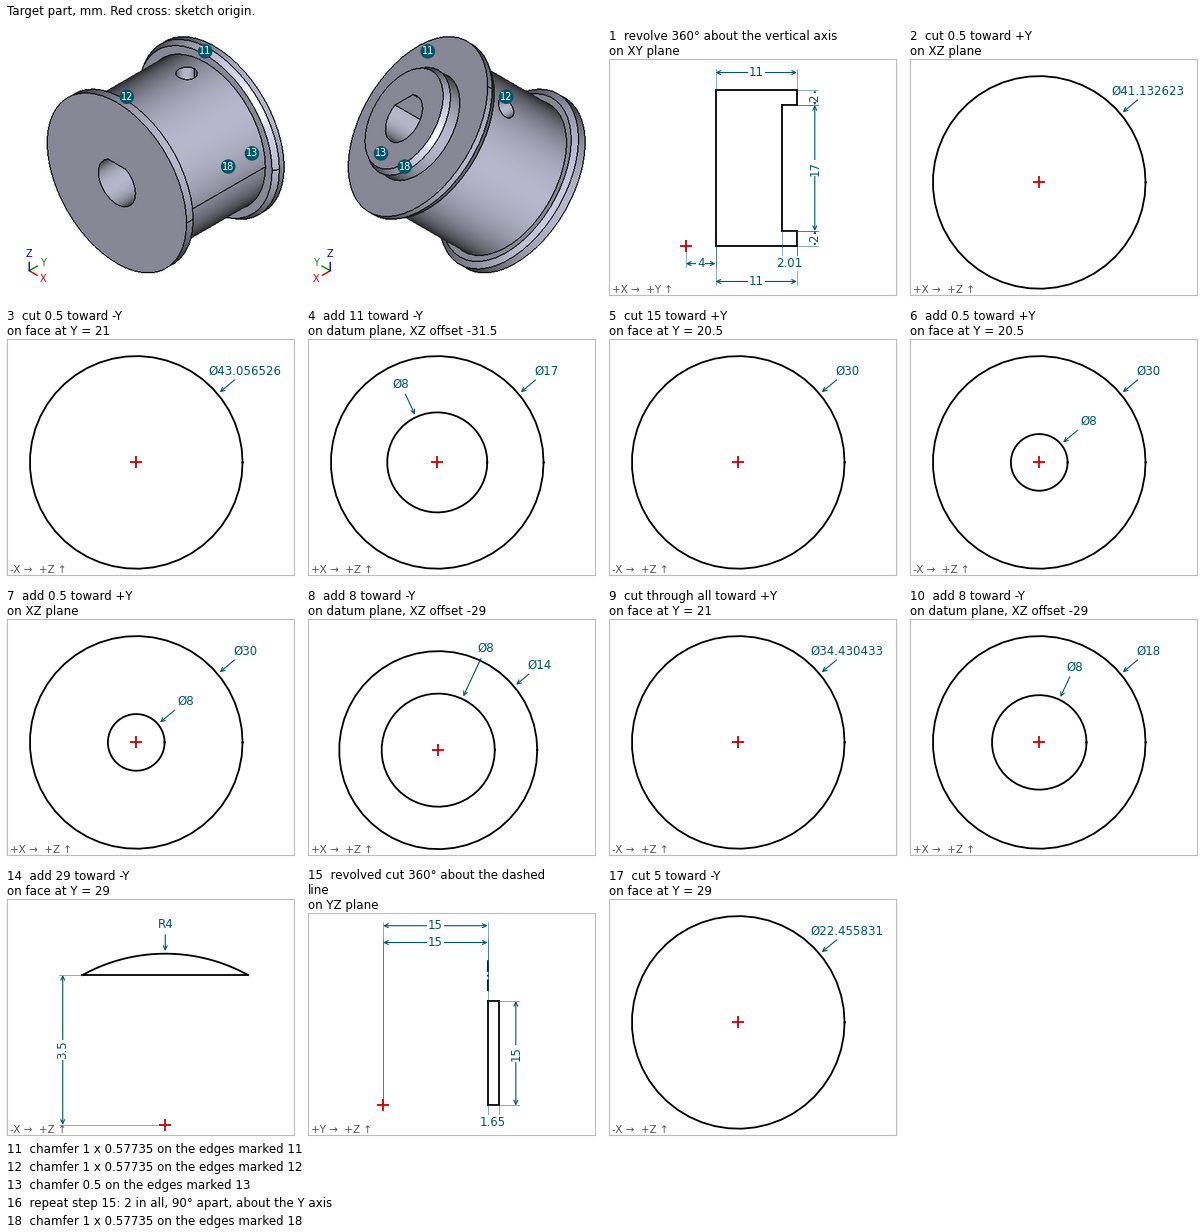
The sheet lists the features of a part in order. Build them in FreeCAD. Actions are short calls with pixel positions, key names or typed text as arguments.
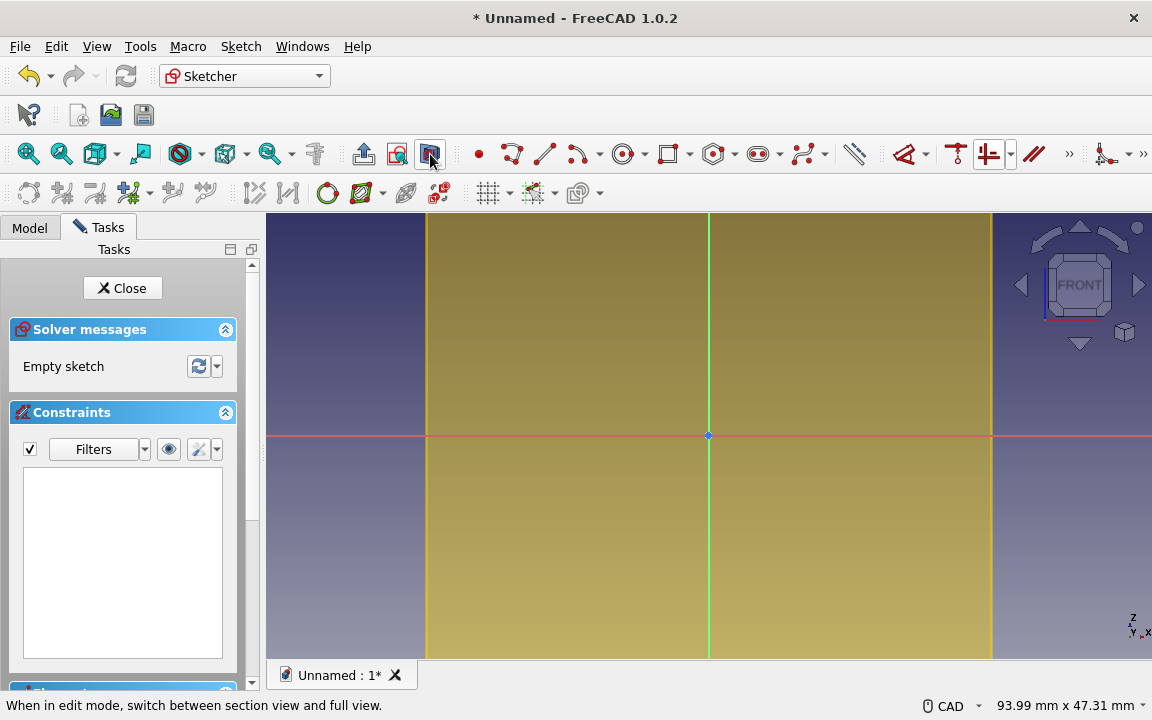
scroll(792, 436, up, 3)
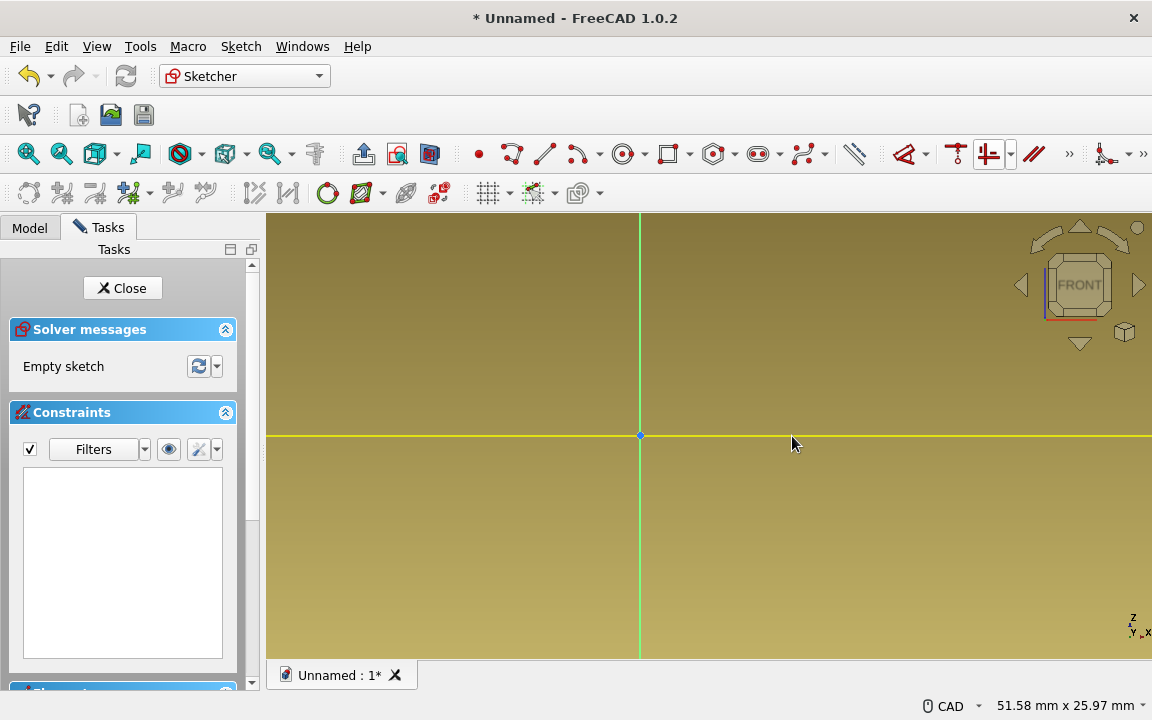
click(622, 154)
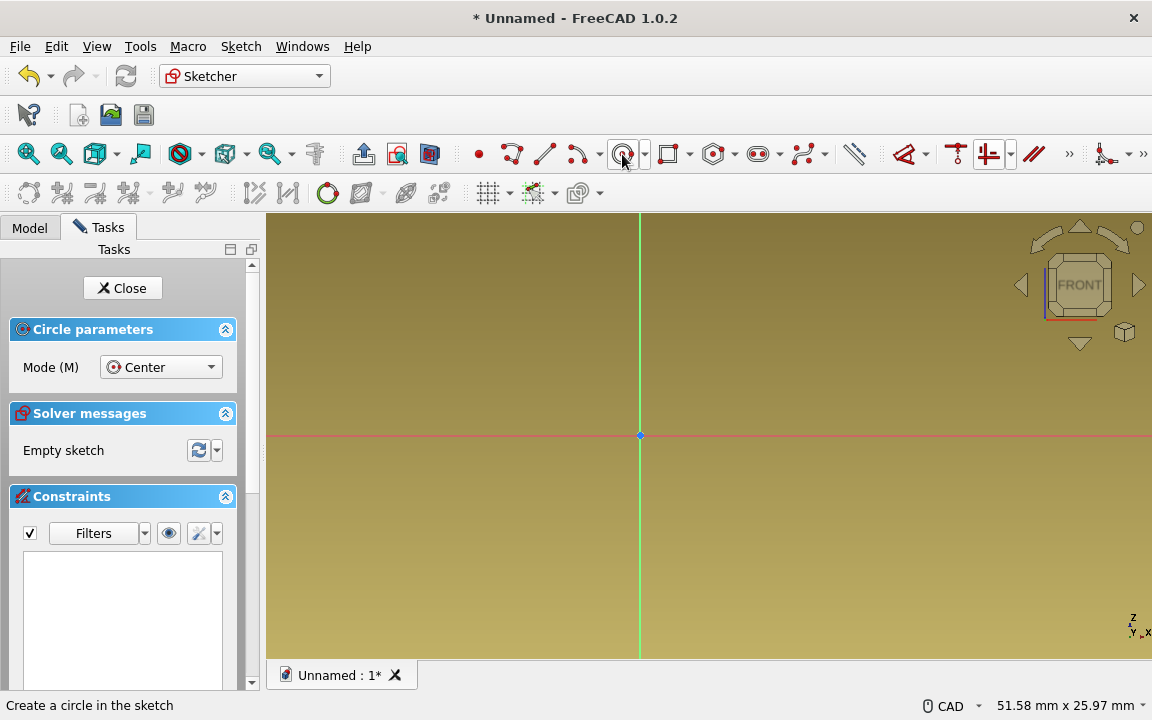
click(640, 436)
move(743, 332)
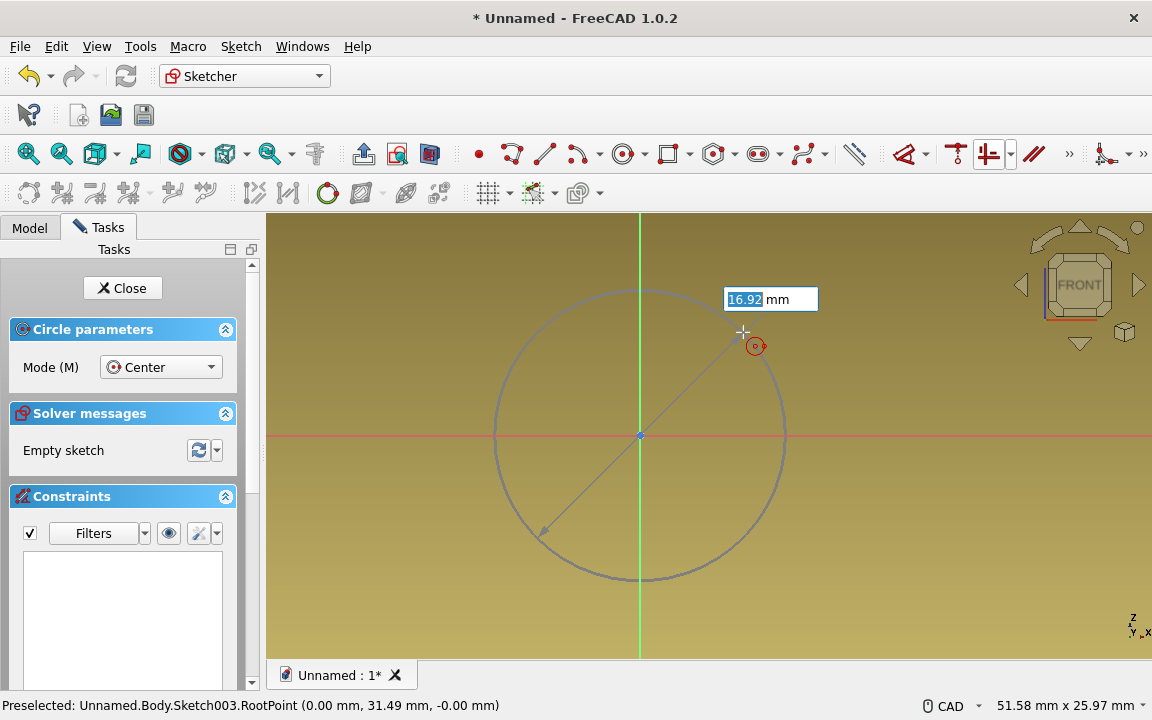
text(17)
key(Return)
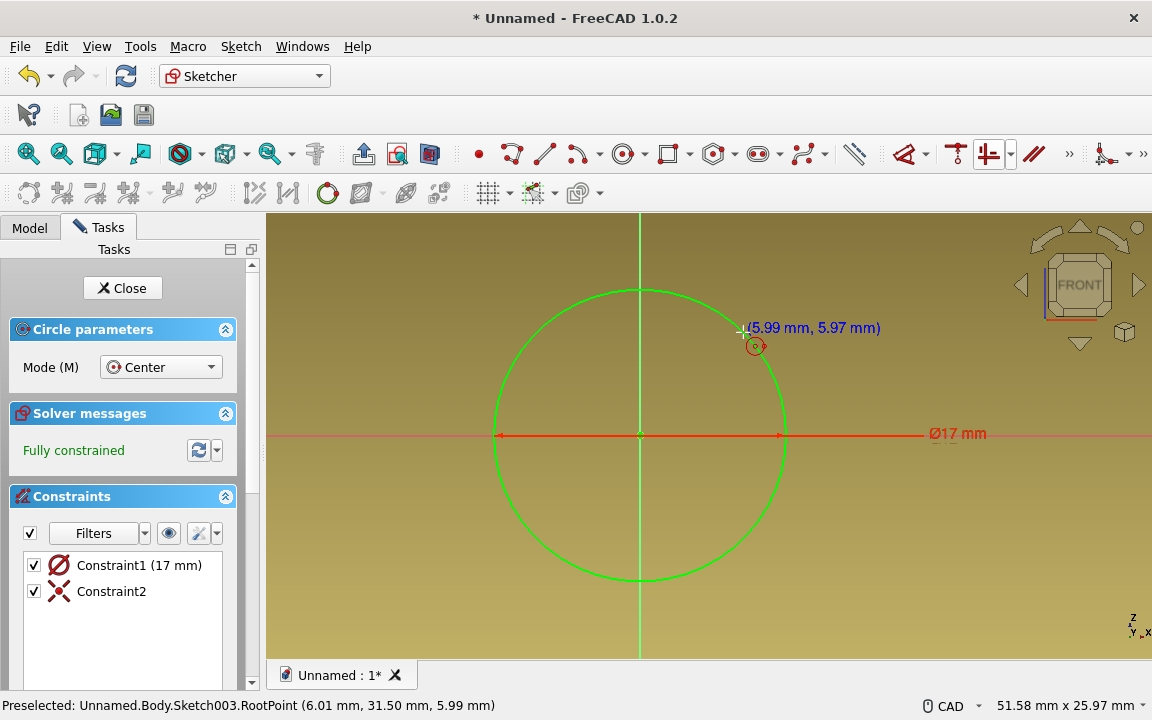
click(640, 436)
move(689, 387)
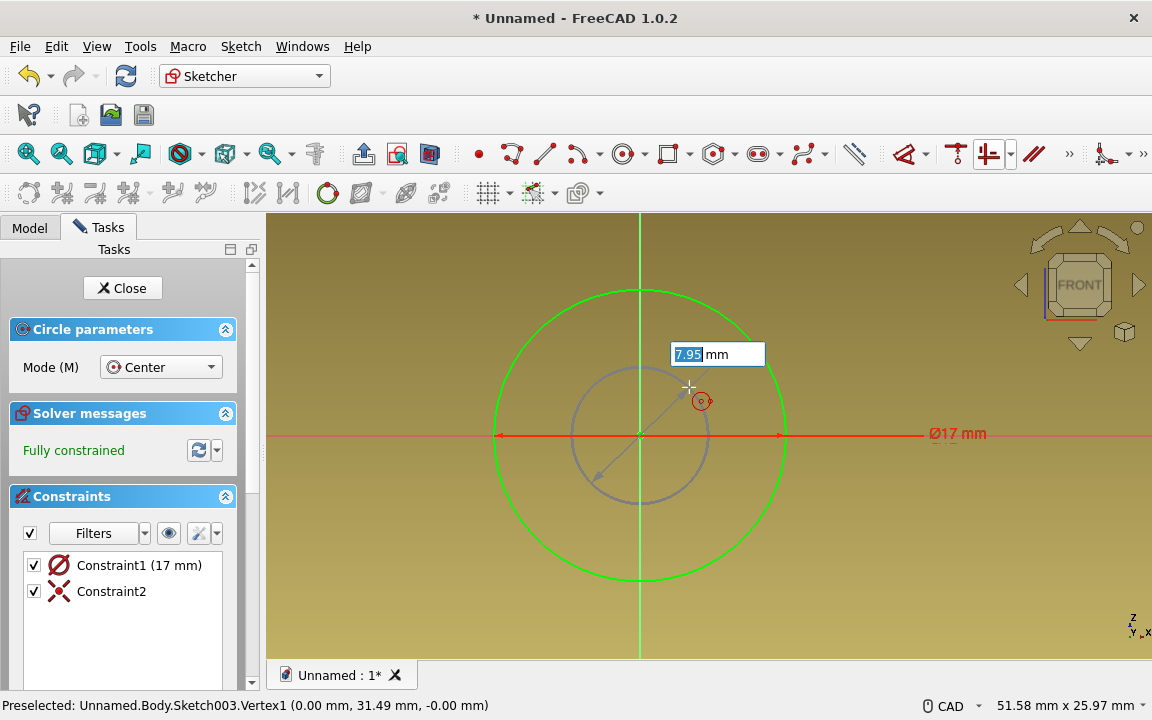
text(8)
key(Return)
key(Escape)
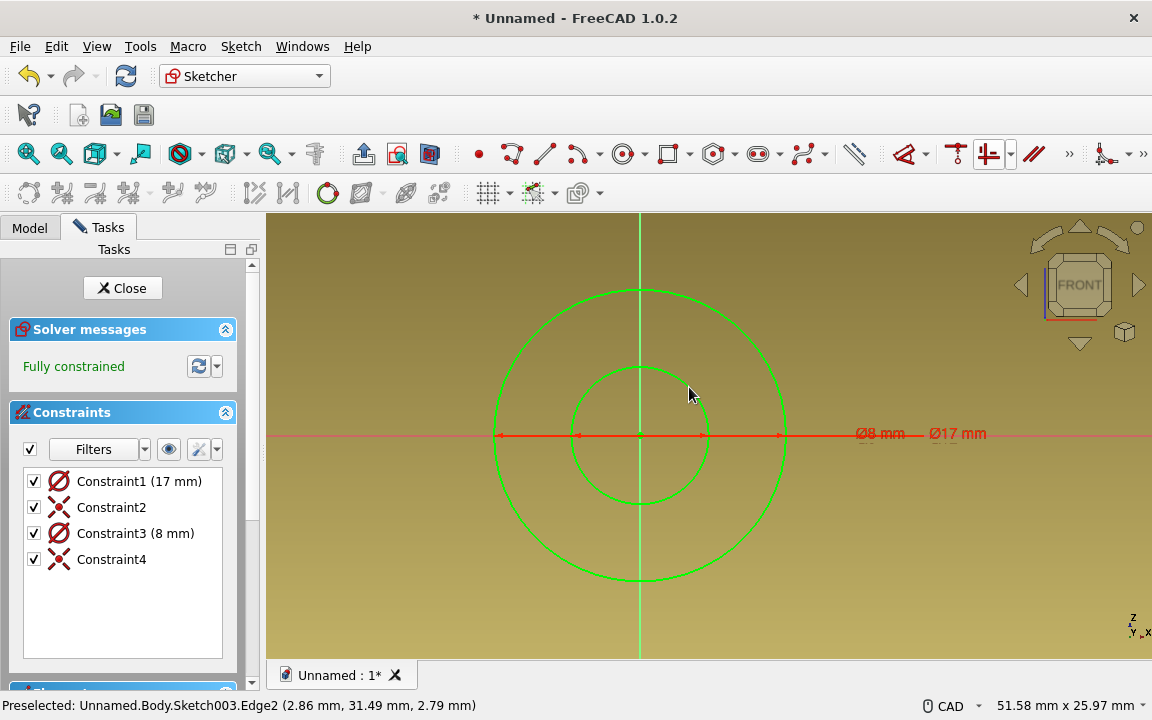
click(123, 288)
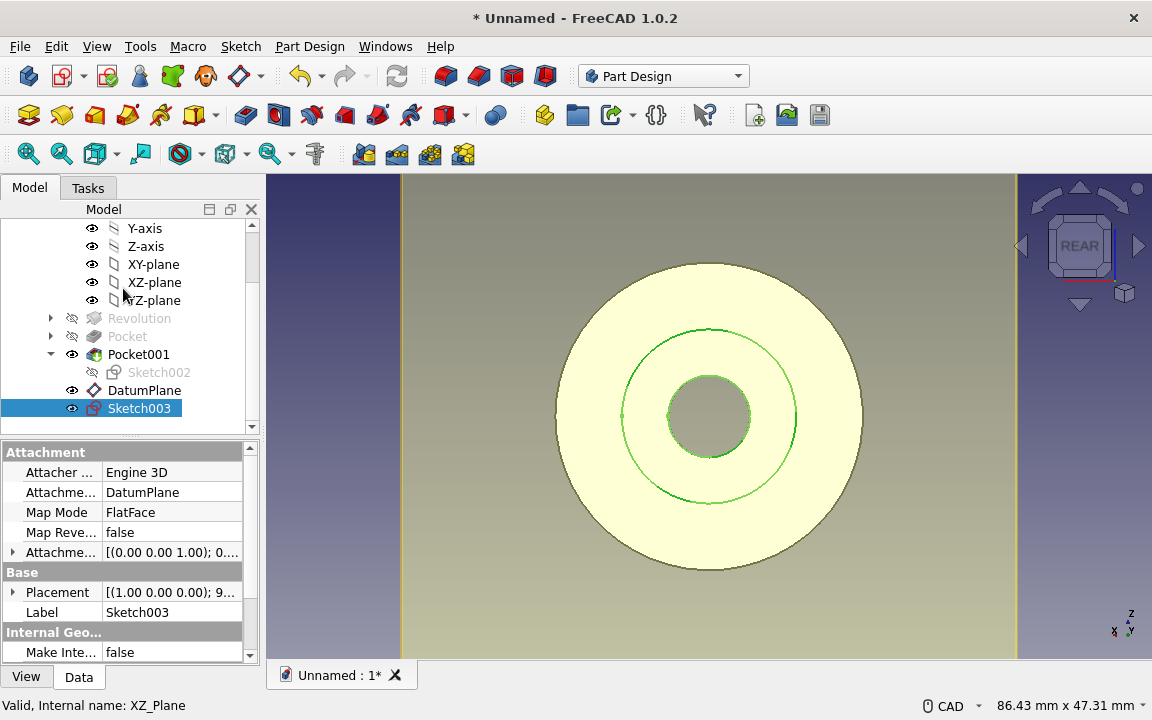
click(29, 116)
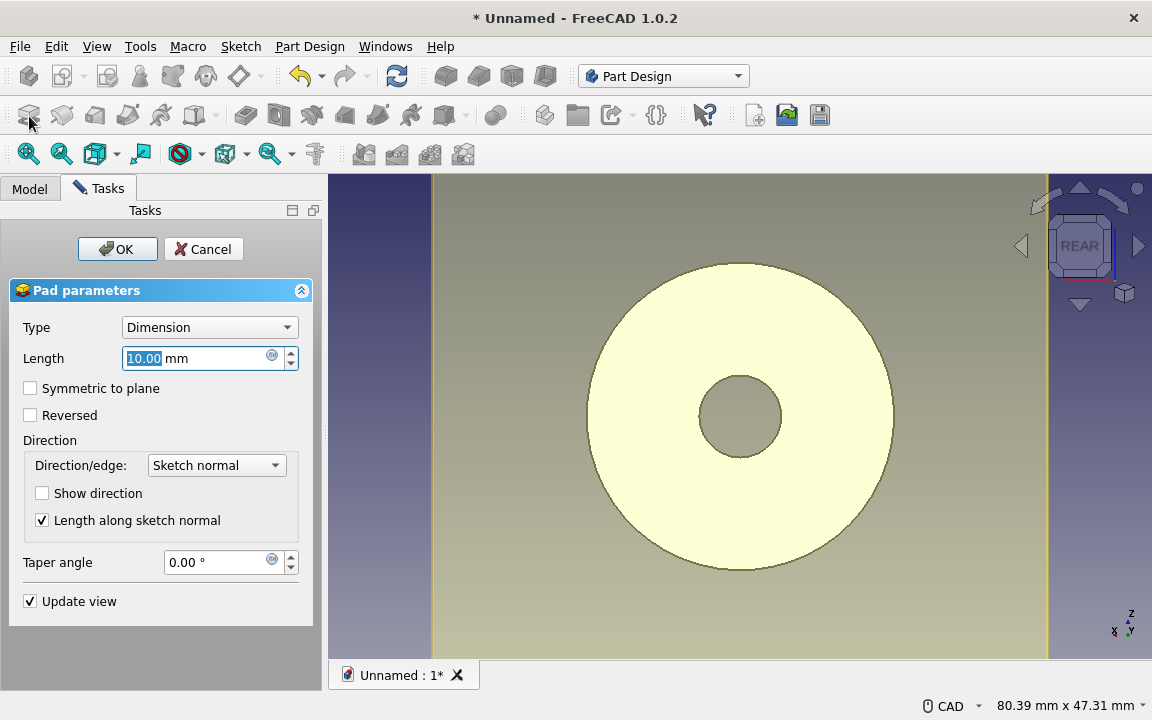
text(11)
key(Tab)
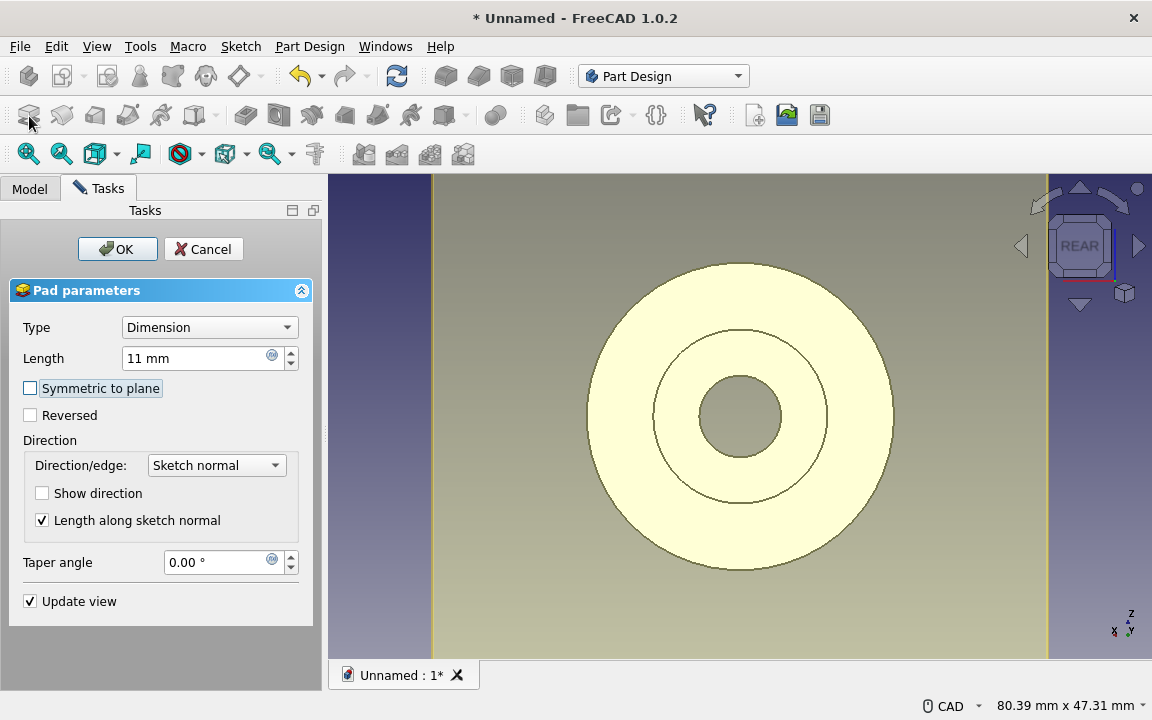
click(118, 249)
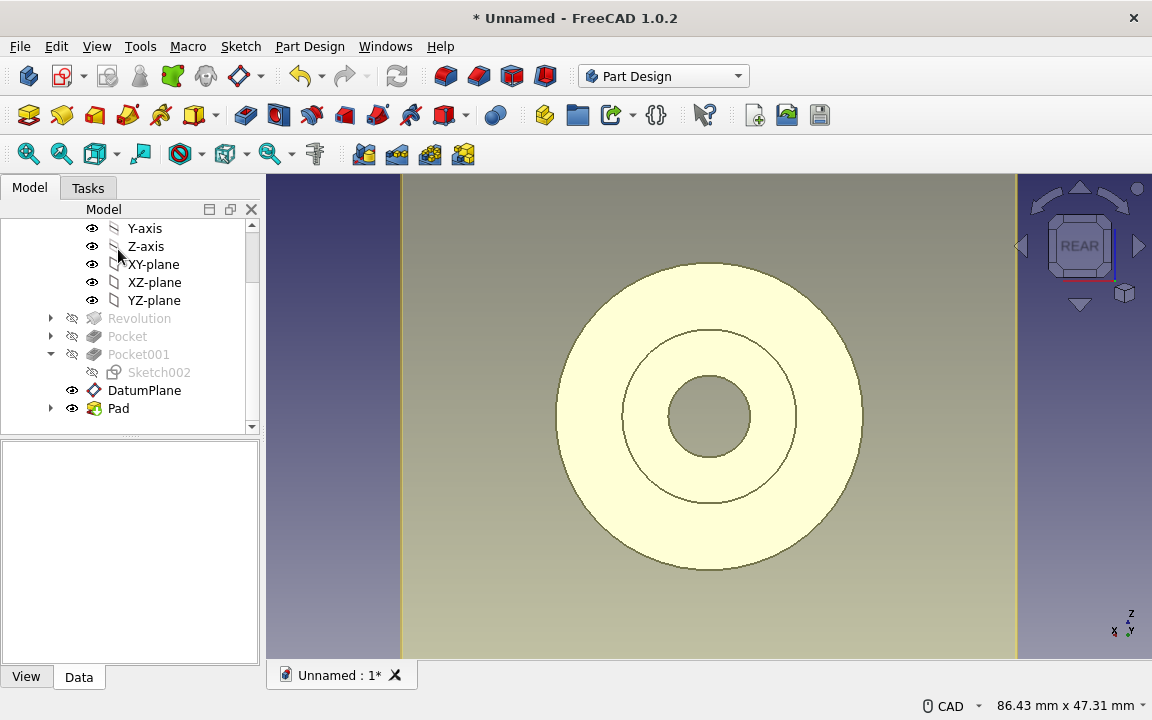
click(117, 390)
key(space)